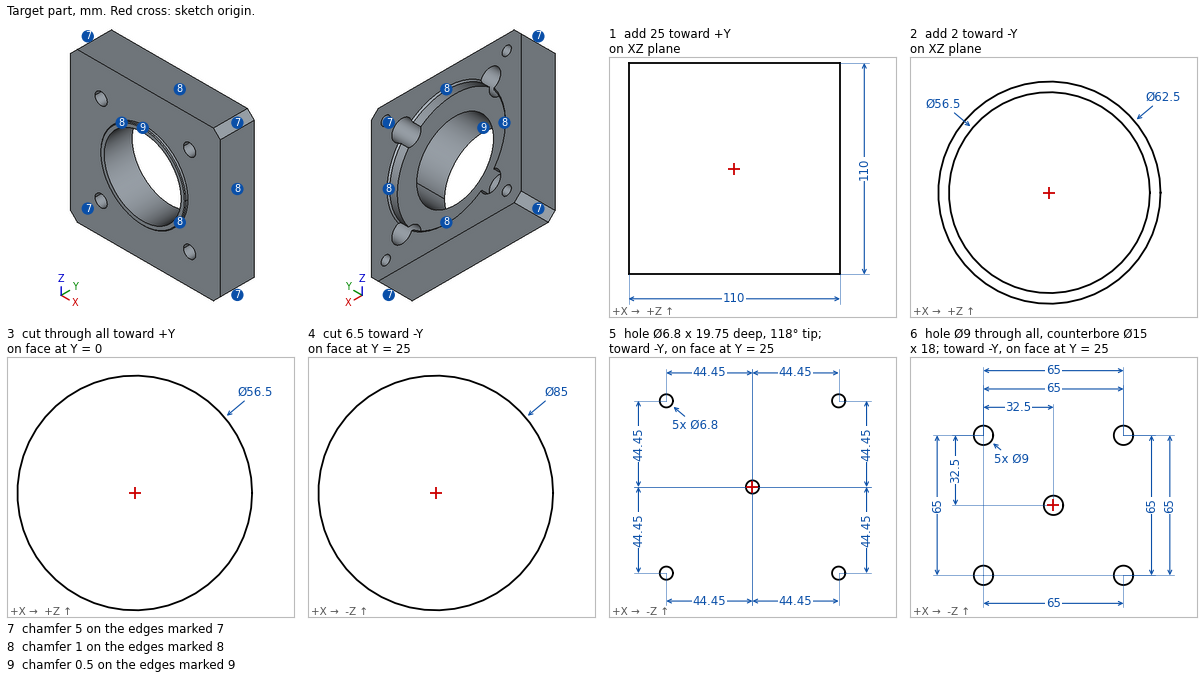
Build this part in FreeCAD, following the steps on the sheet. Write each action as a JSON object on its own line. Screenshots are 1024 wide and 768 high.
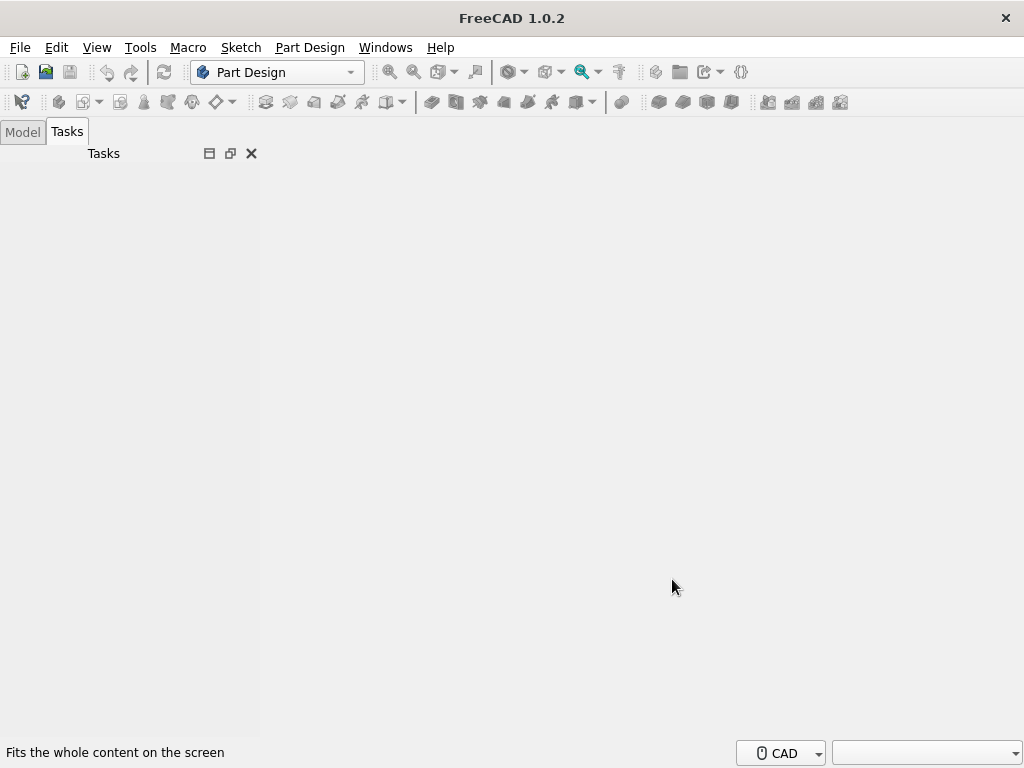
{"action": "left_click", "coordinate": [22, 72]}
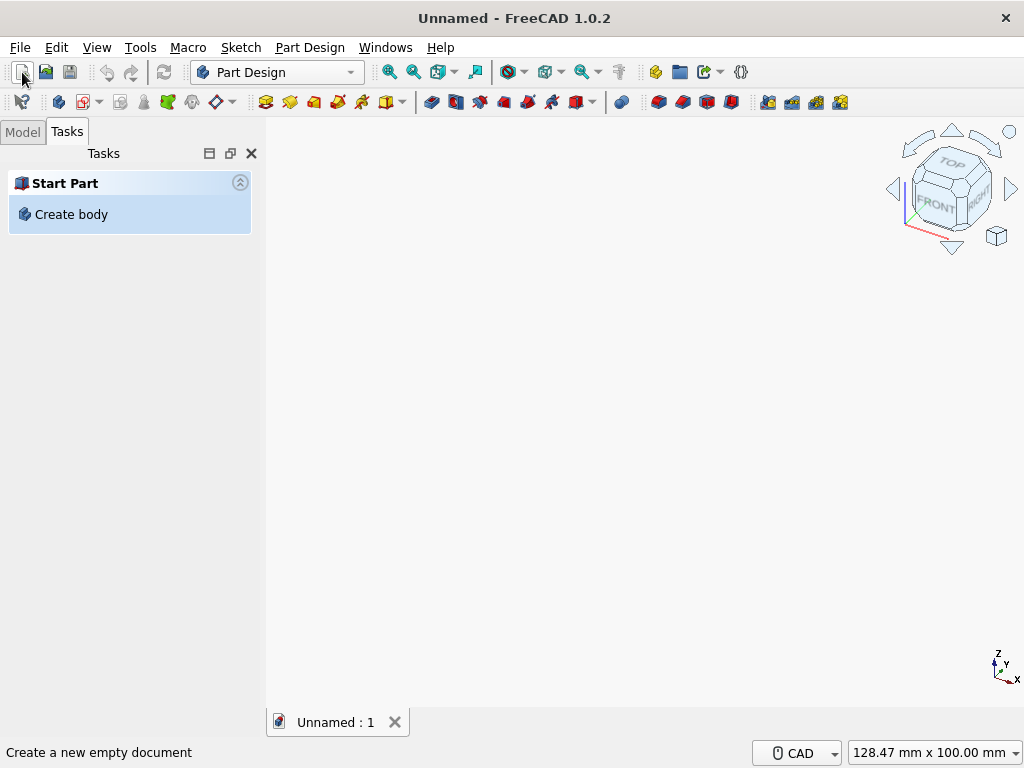
{"action": "left_click", "coordinate": [84, 102]}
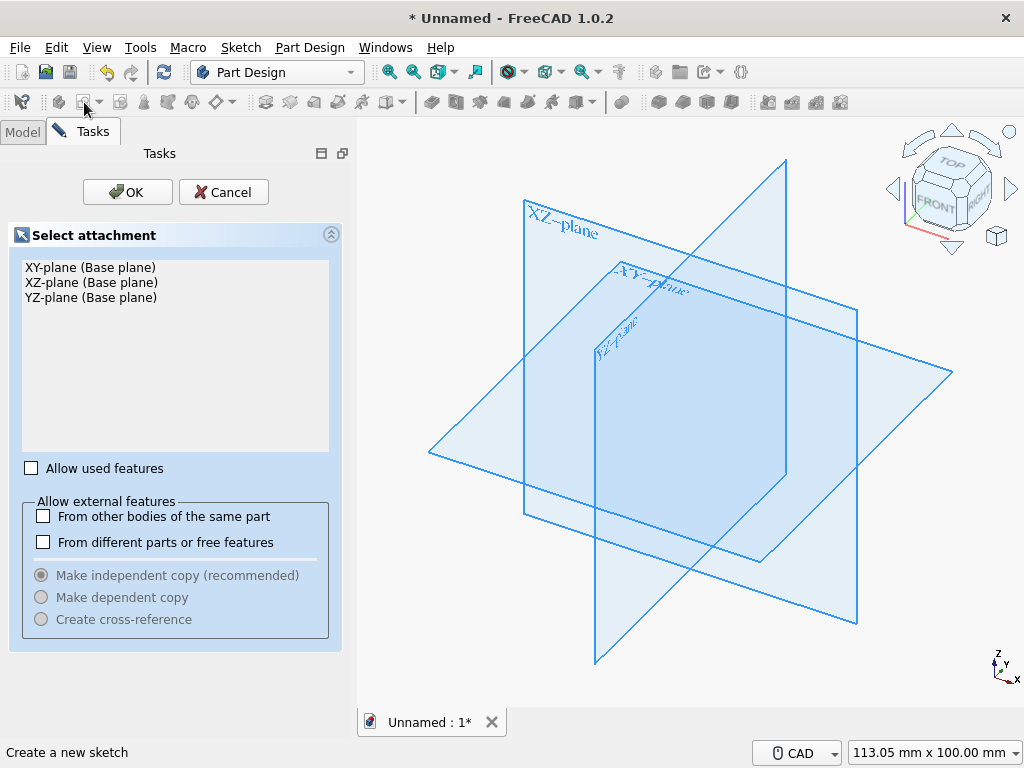
{"action": "left_click", "coordinate": [82, 282]}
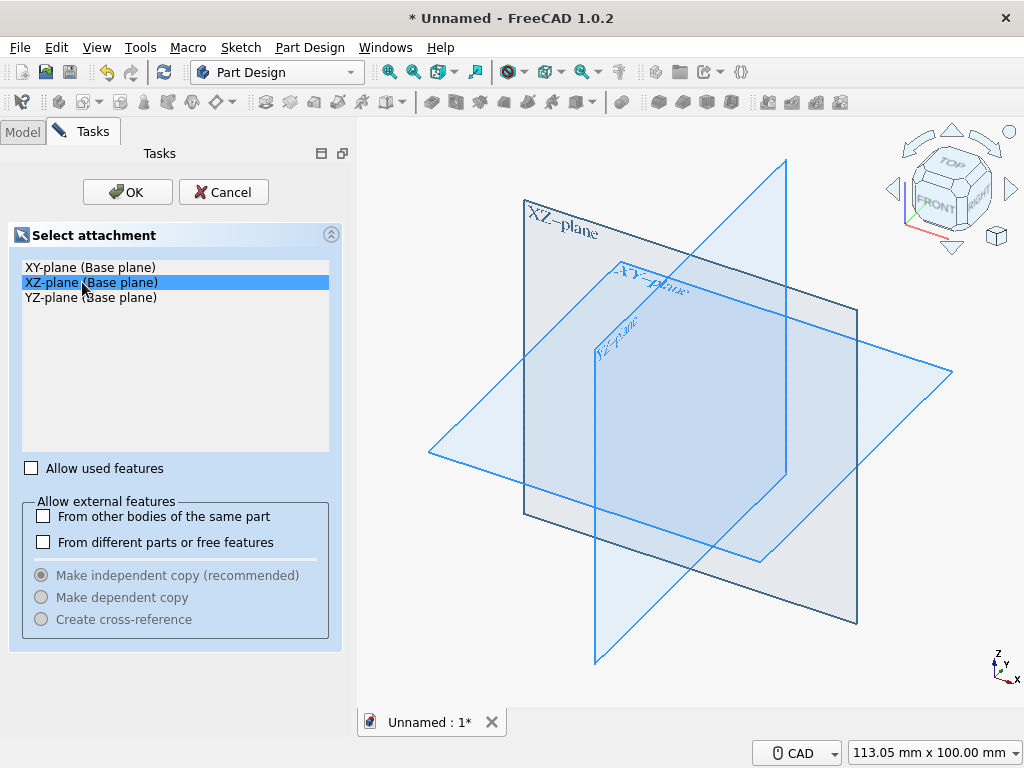
{"action": "left_click", "coordinate": [128, 192]}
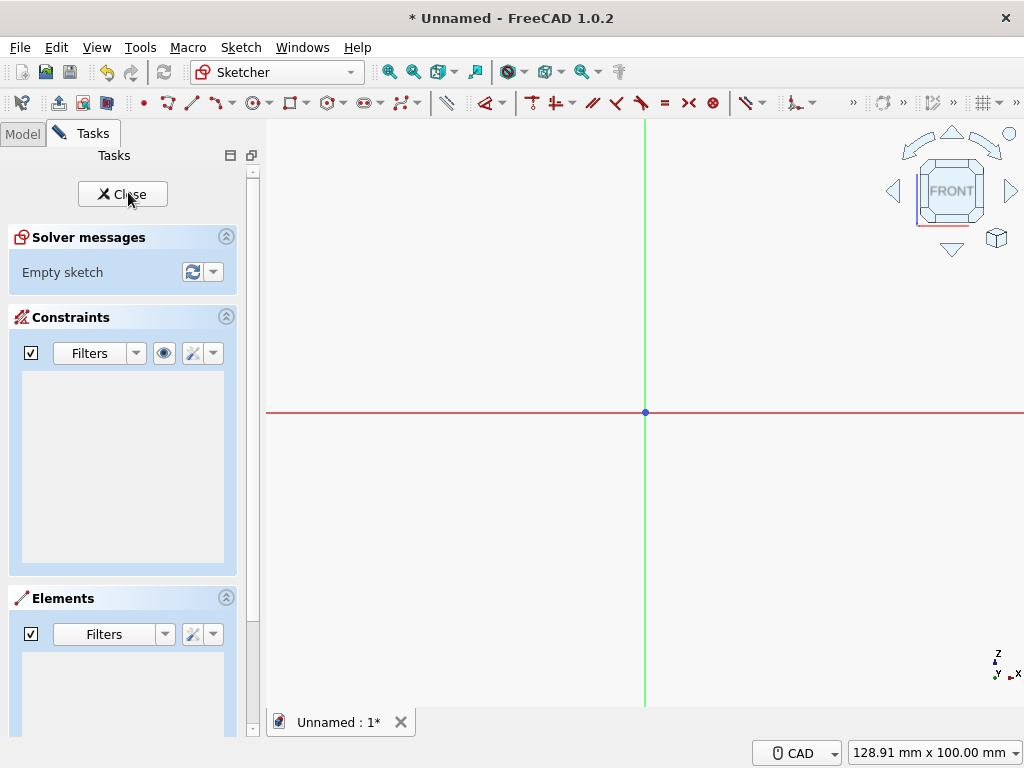
{"action": "scroll", "coordinate": [493, 413], "scroll_direction": "down", "scroll_amount": 3}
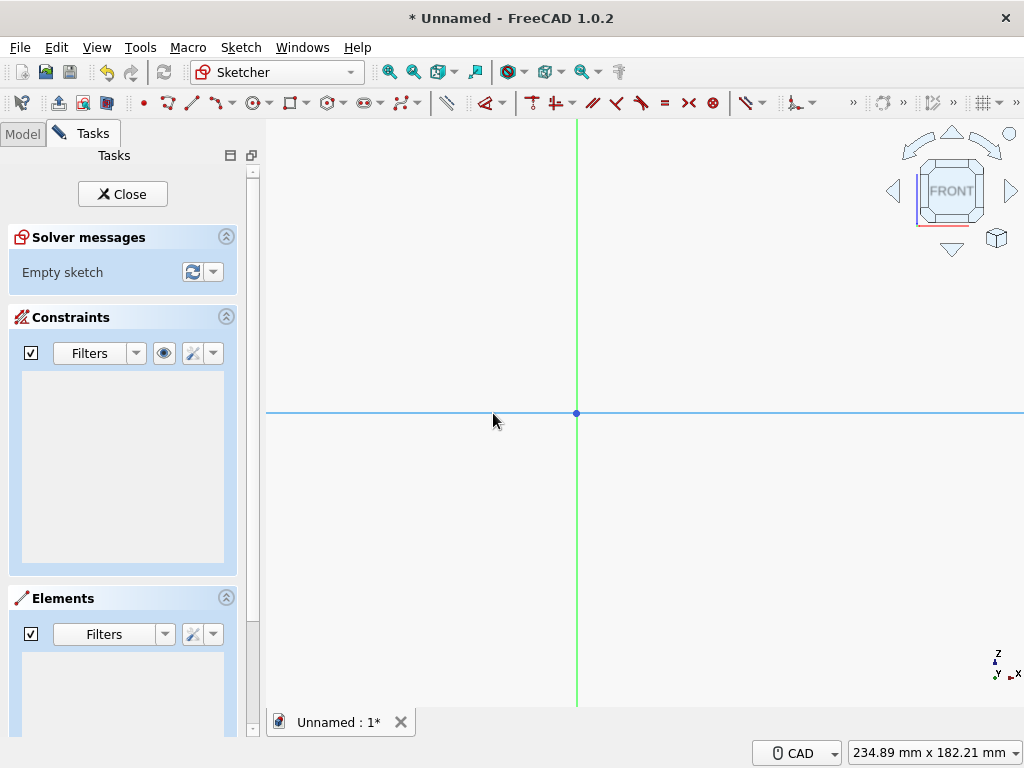
{"action": "left_click", "coordinate": [308, 104]}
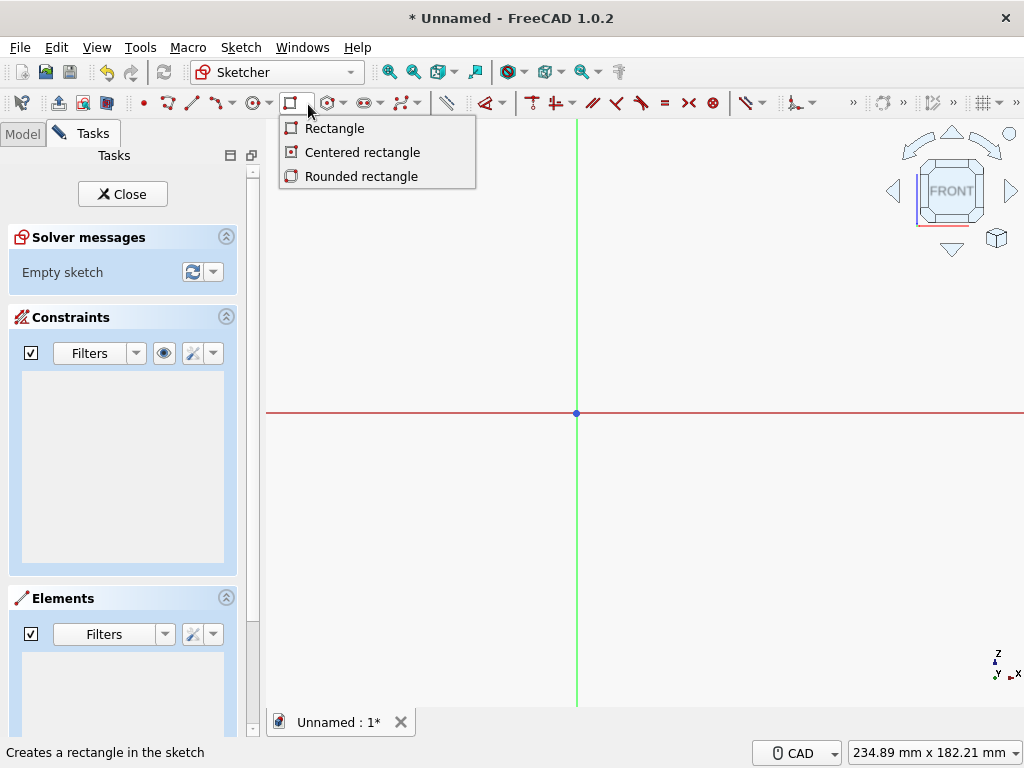
{"action": "left_click", "coordinate": [378, 152]}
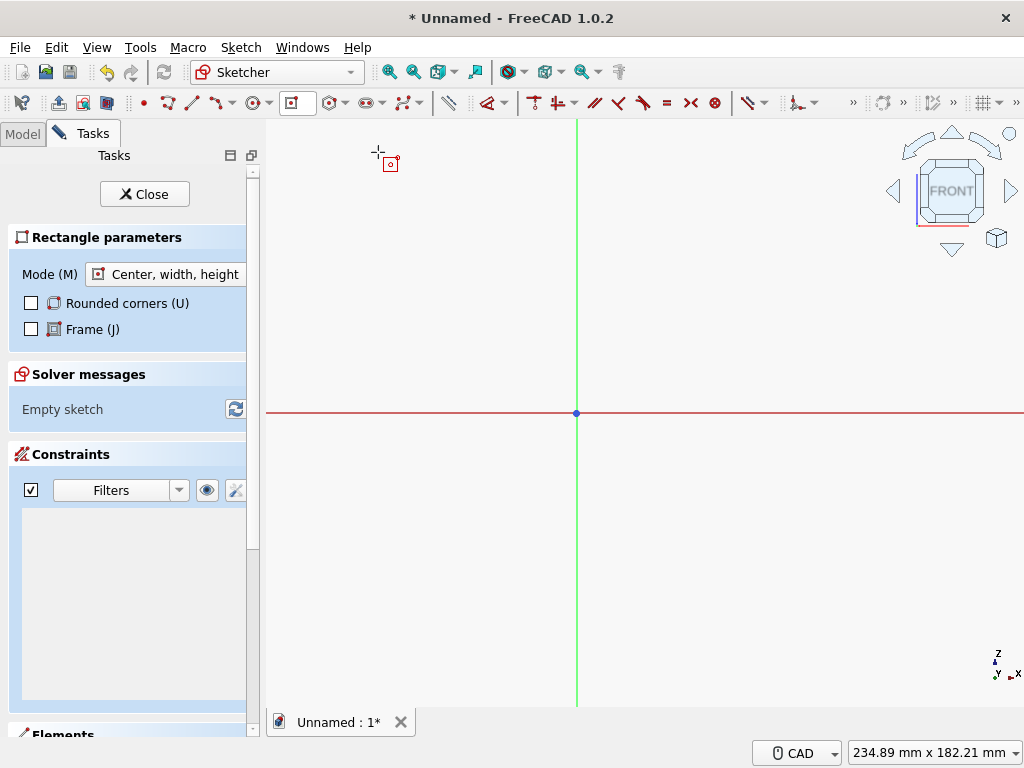
{"action": "left_click", "coordinate": [577, 413]}
{"action": "left_click", "coordinate": [754, 236]}
{"action": "key", "text": "Escape"}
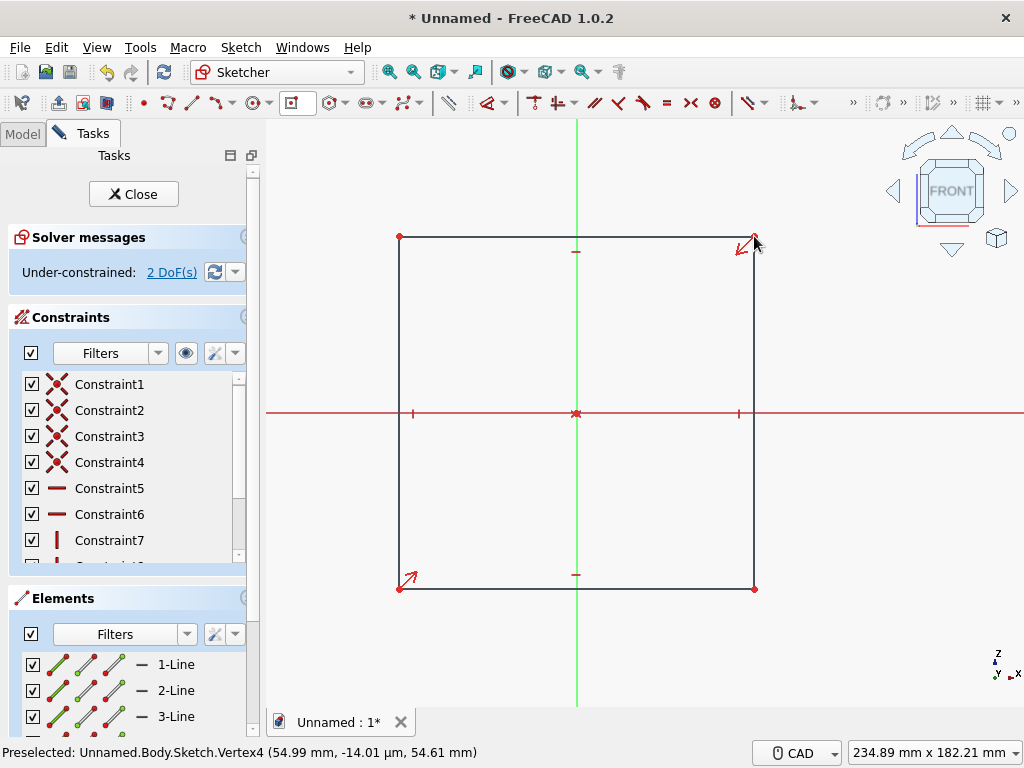
{"action": "left_click", "coordinate": [488, 104]}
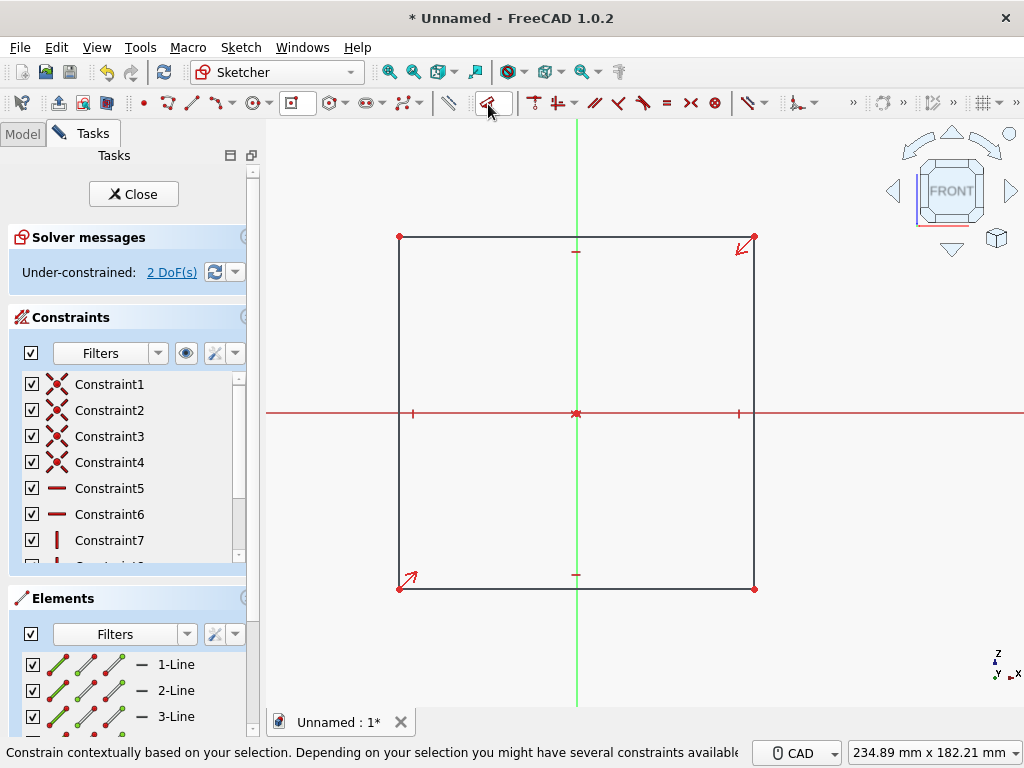
{"action": "left_click", "coordinate": [506, 589]}
{"action": "left_click", "coordinate": [495, 623]}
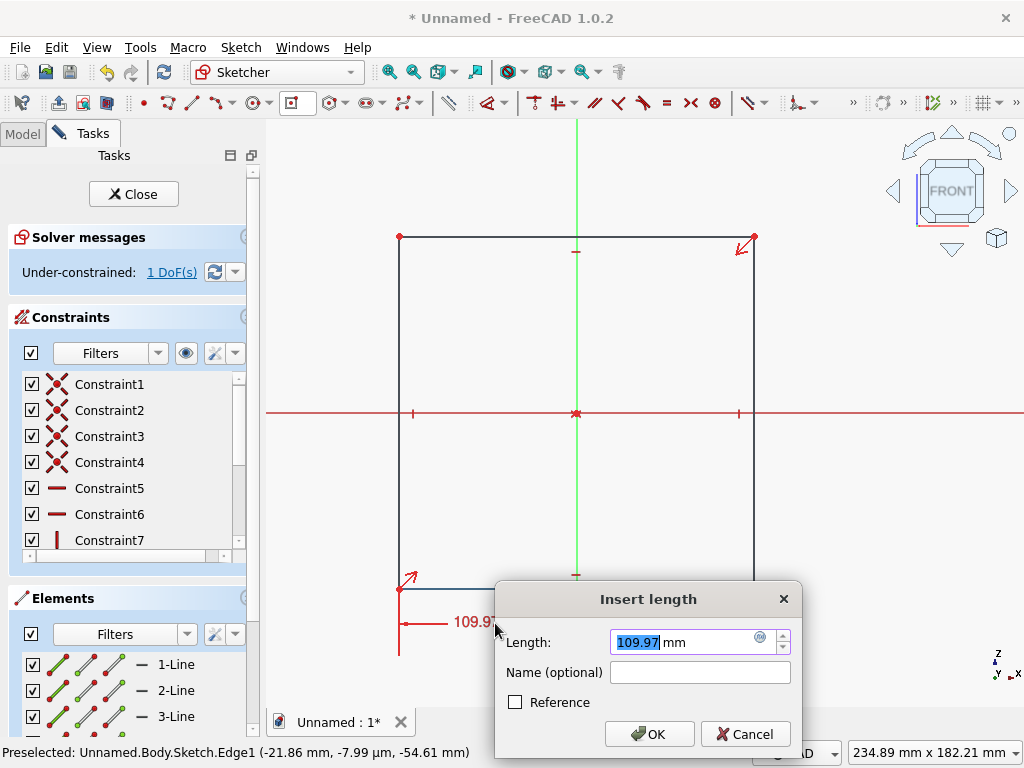
{"action": "type", "text": "110"}
{"action": "key", "text": "Return"}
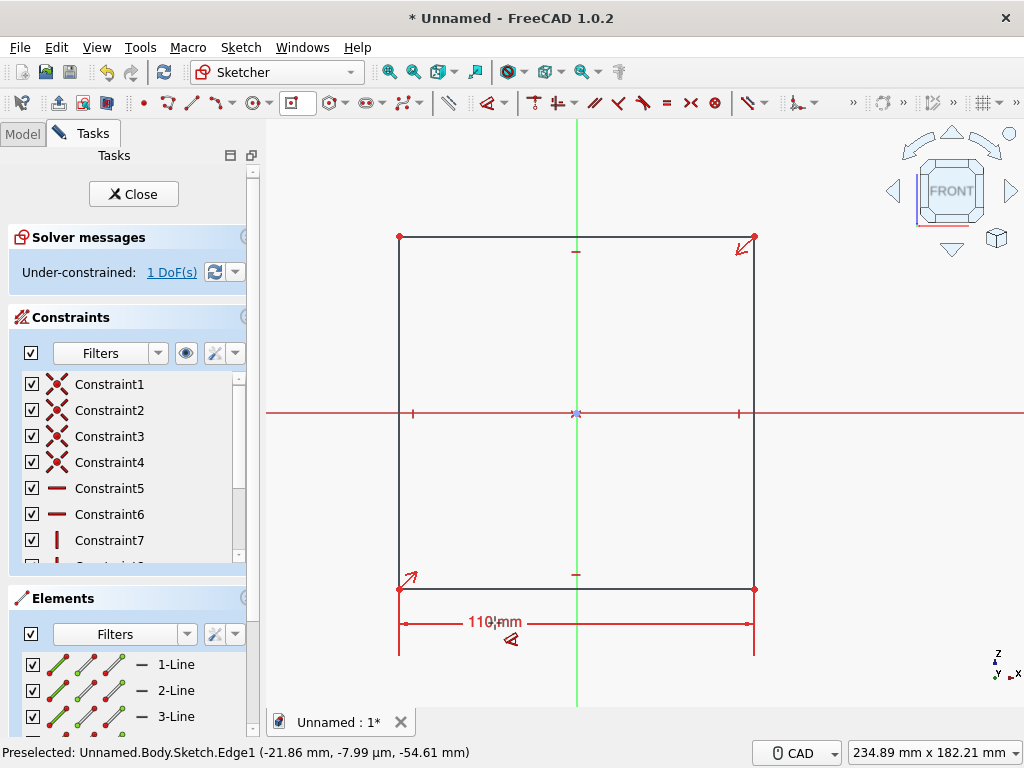
{"action": "left_click", "coordinate": [754, 484]}
{"action": "left_click", "coordinate": [788, 332]}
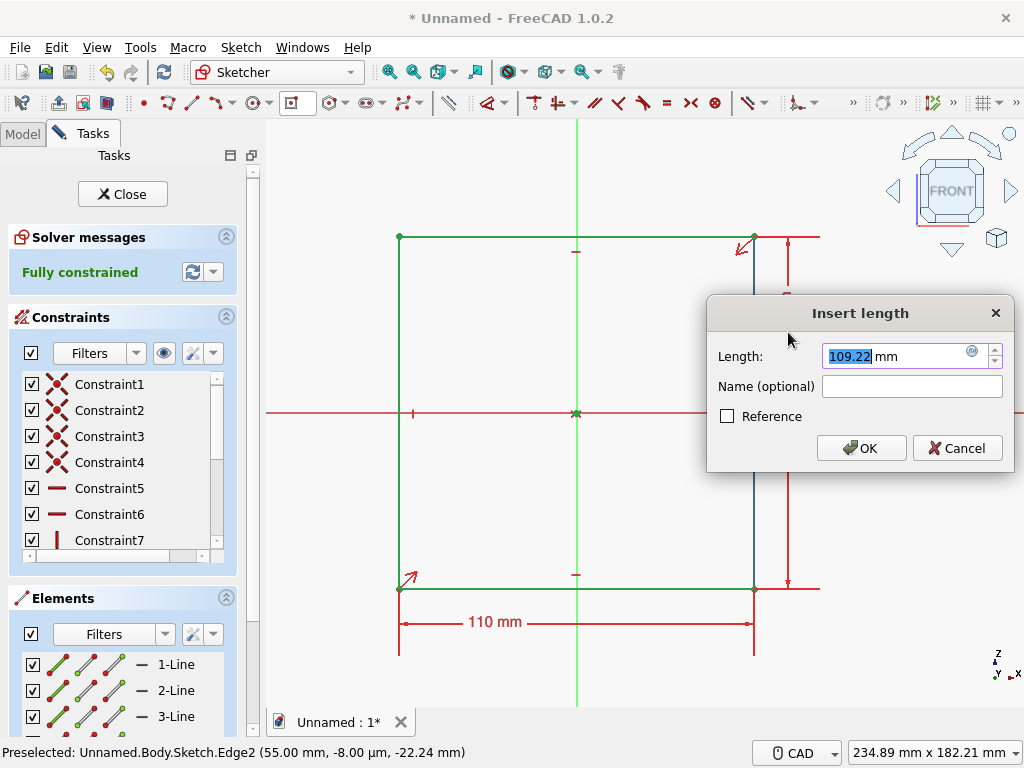
{"action": "type", "text": "110"}
{"action": "key", "text": "Return"}
{"action": "key", "text": "Escape"}